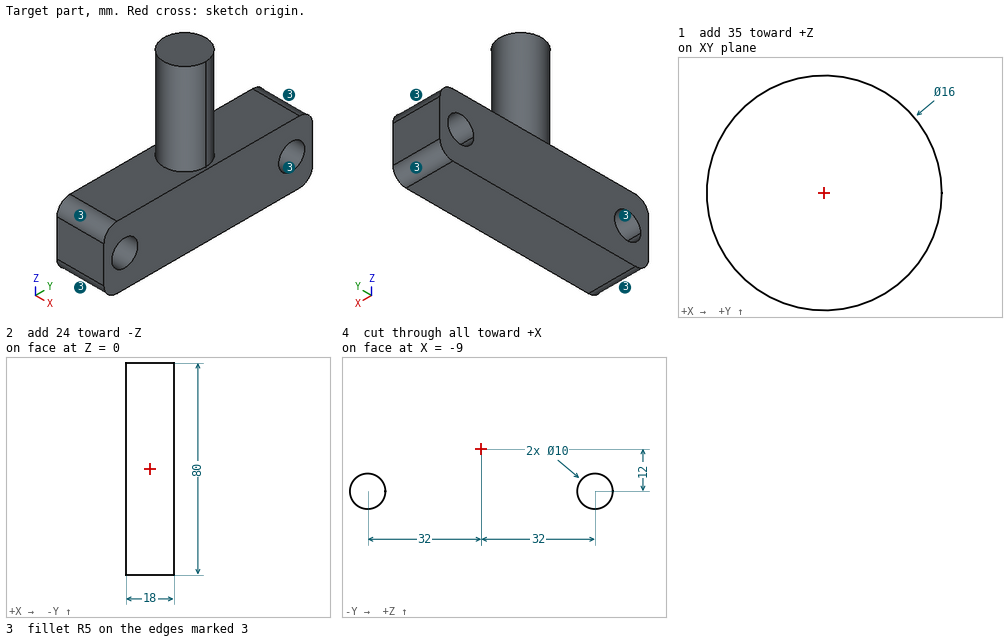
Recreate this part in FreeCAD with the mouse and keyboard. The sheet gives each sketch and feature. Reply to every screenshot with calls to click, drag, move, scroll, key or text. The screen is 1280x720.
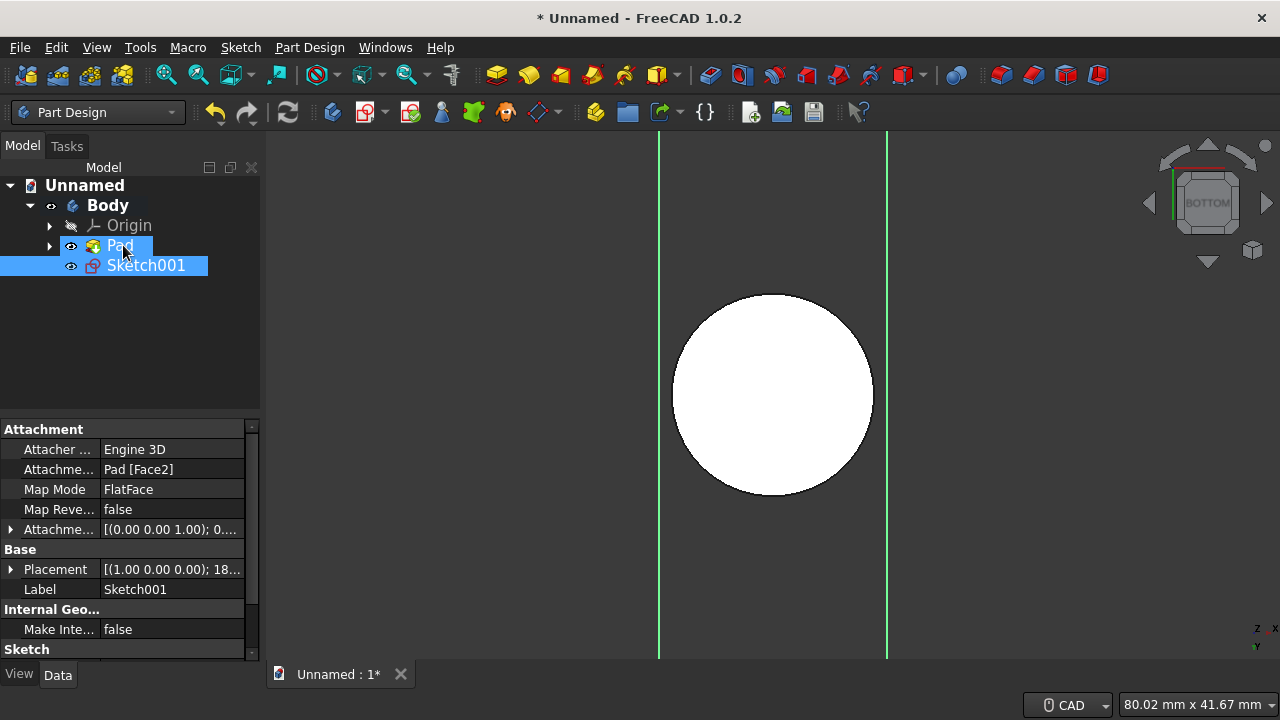
click(498, 76)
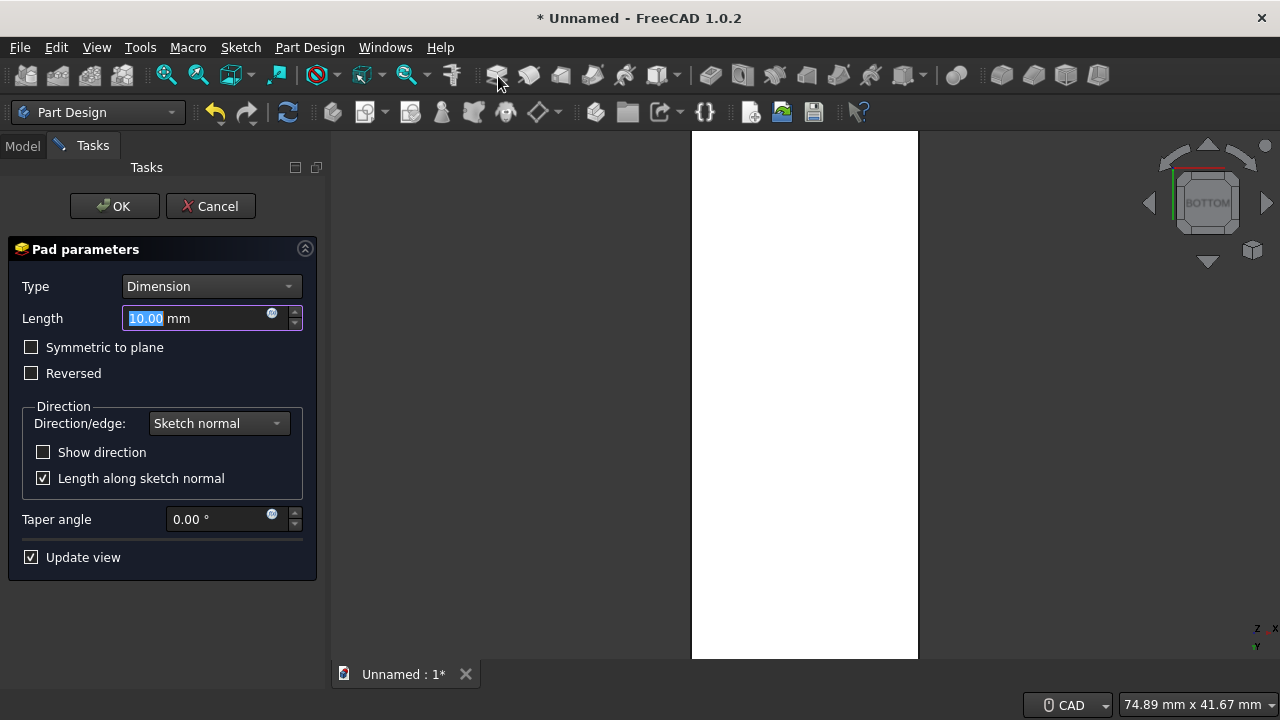
text(24)
key(Tab)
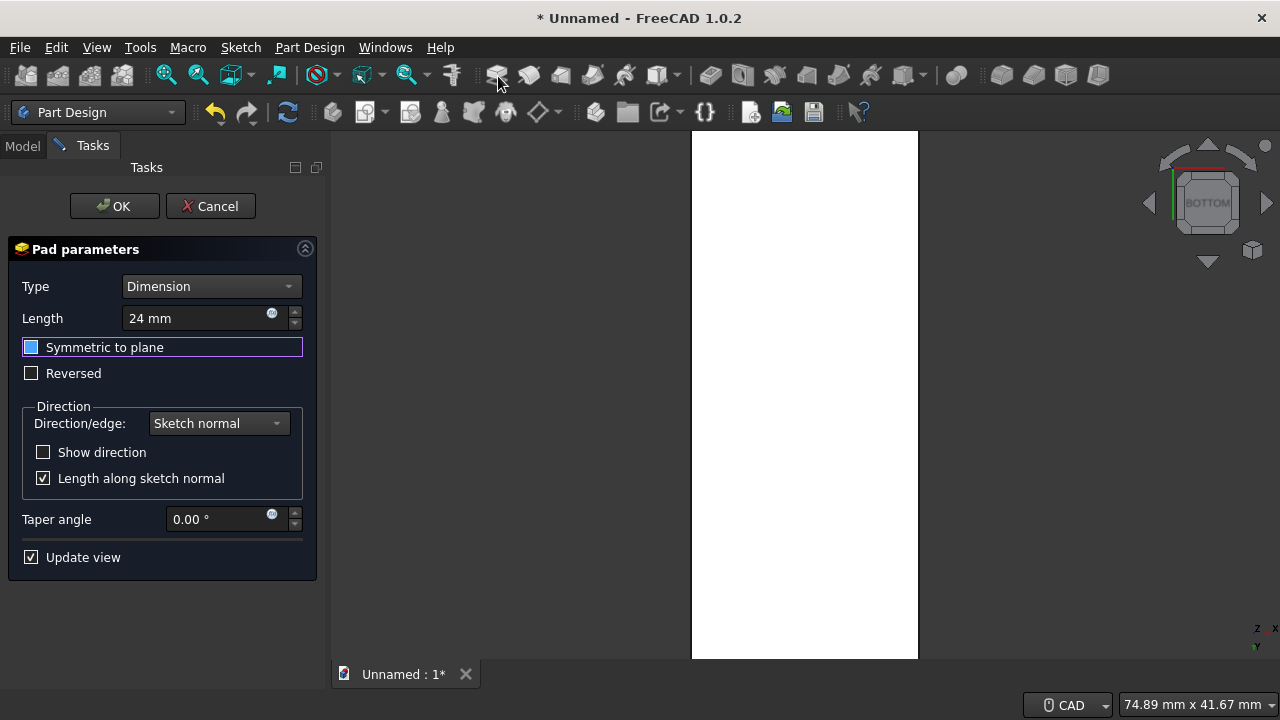
click(115, 206)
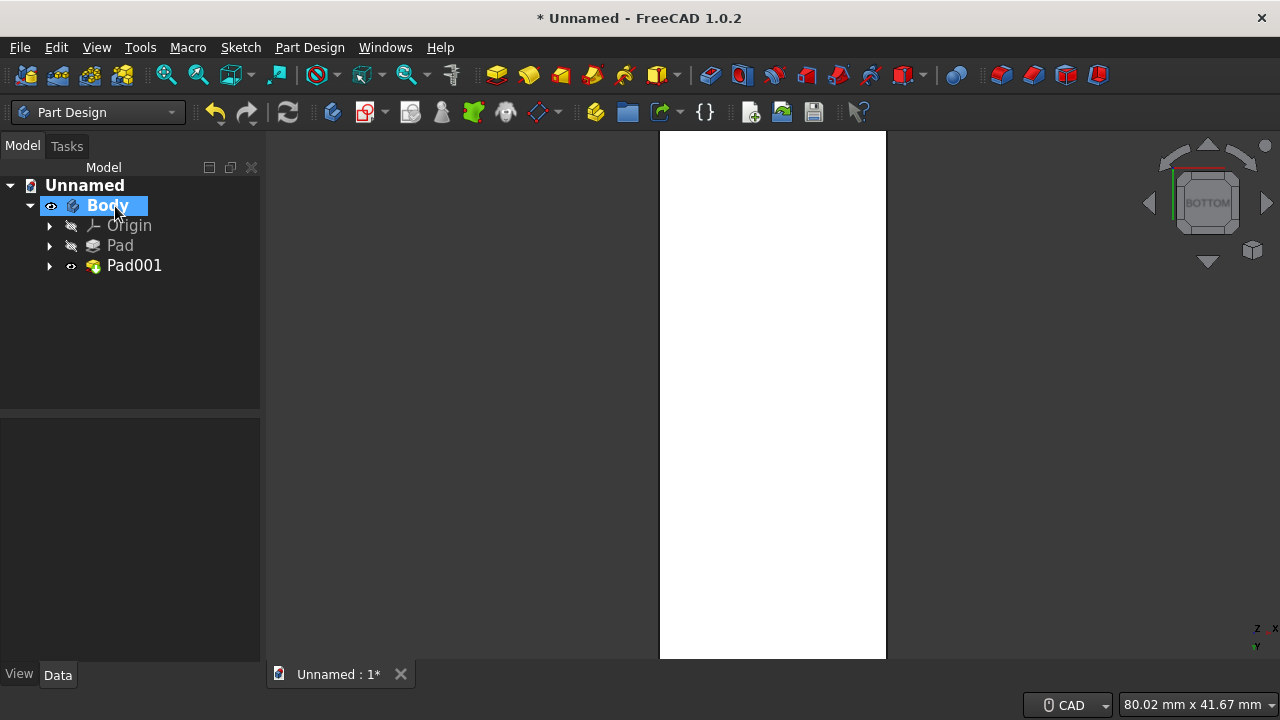
click(168, 76)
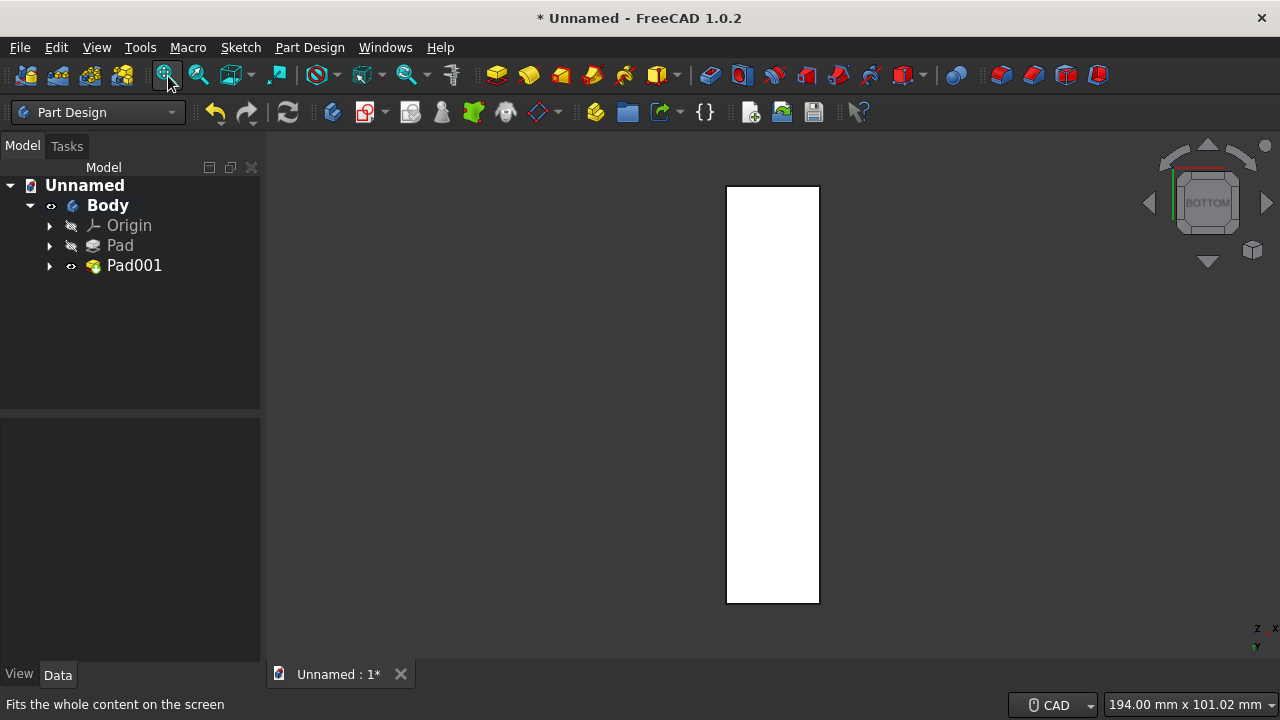
click(773, 603)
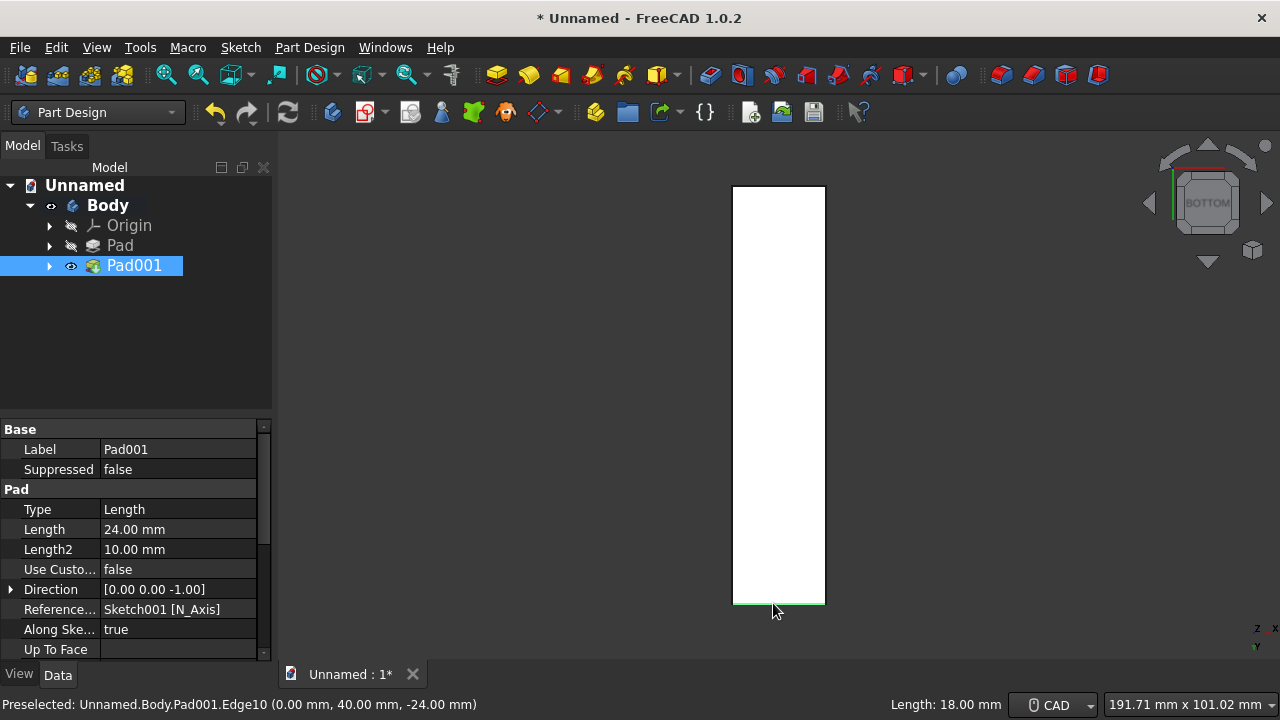
key(0)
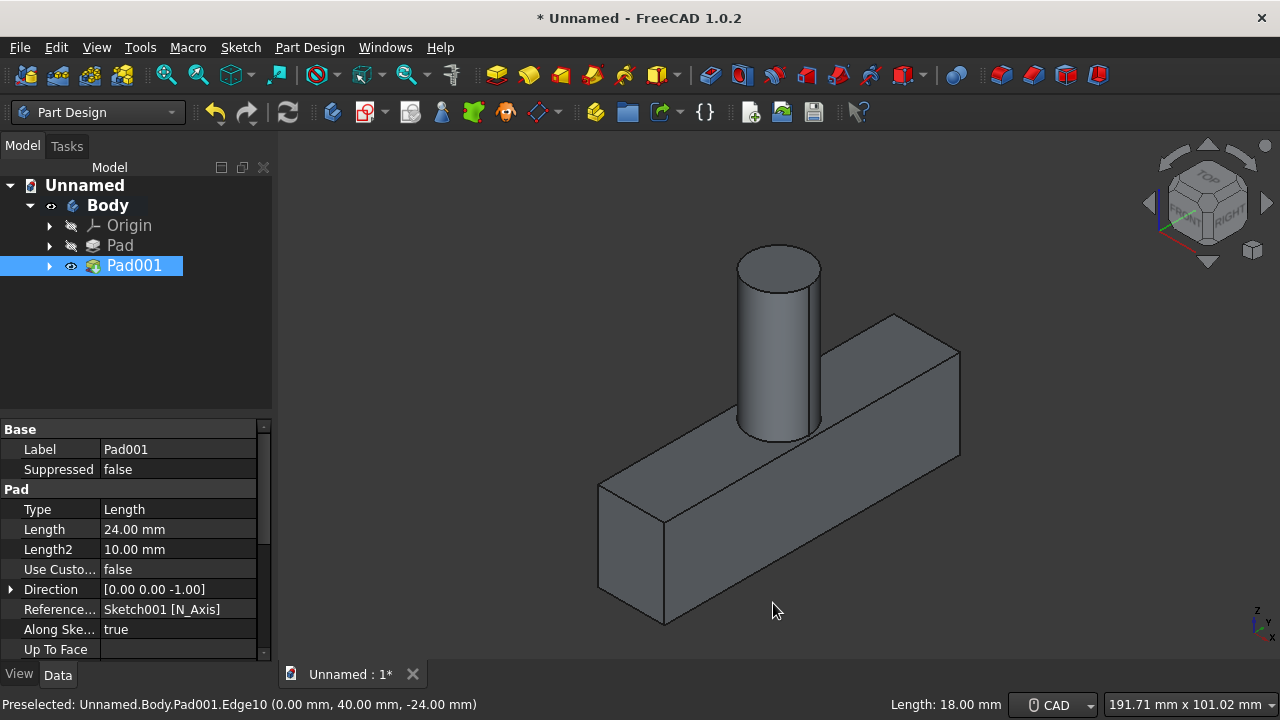
click(631, 503, ctrl)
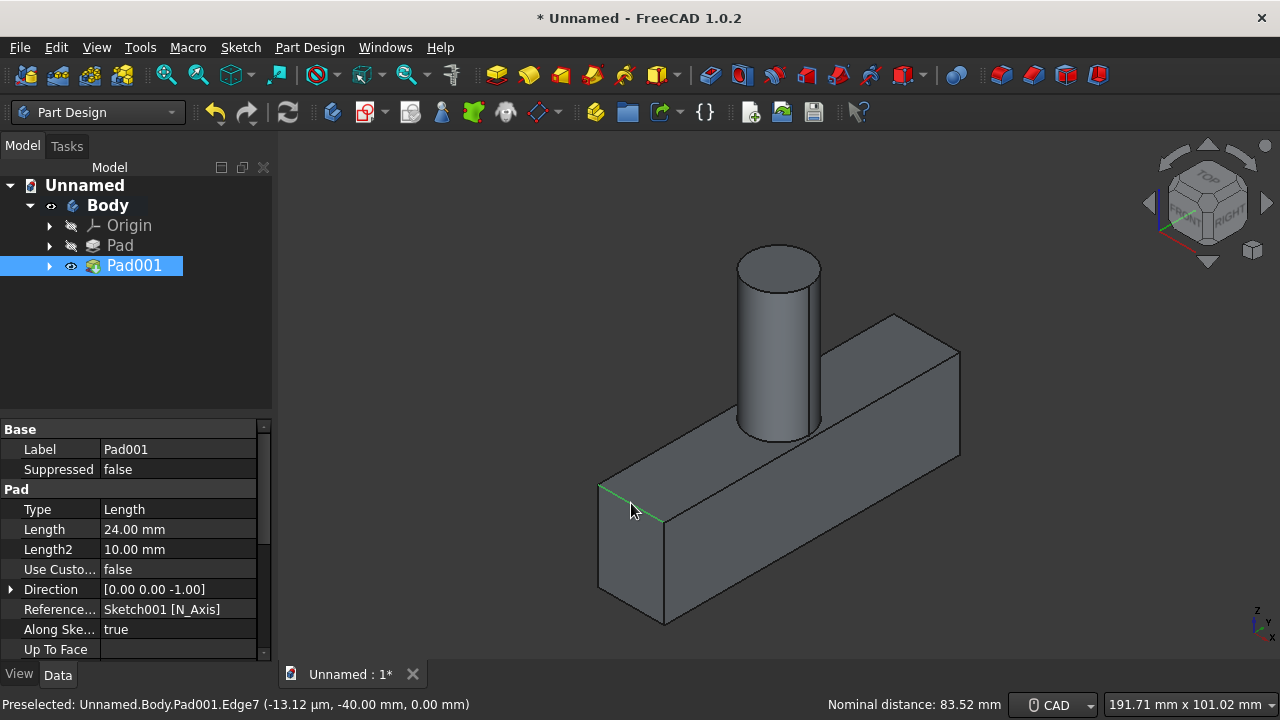
key(2)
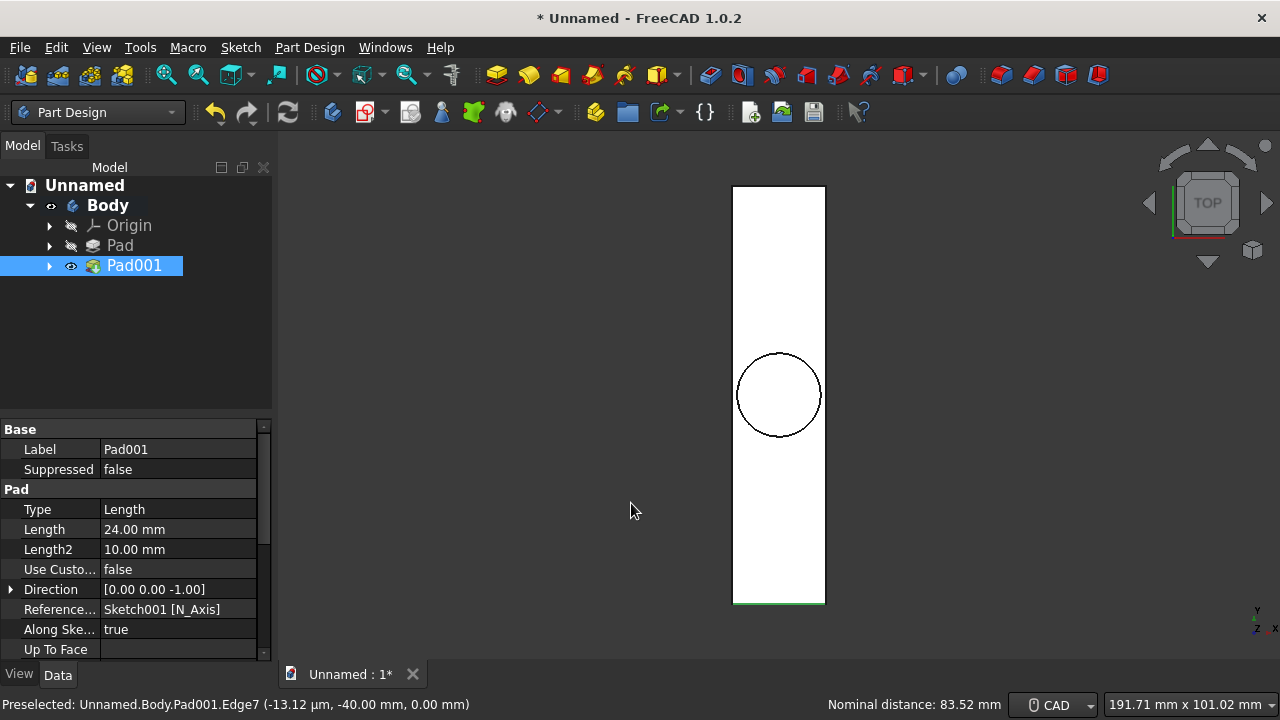
click(779, 185, ctrl)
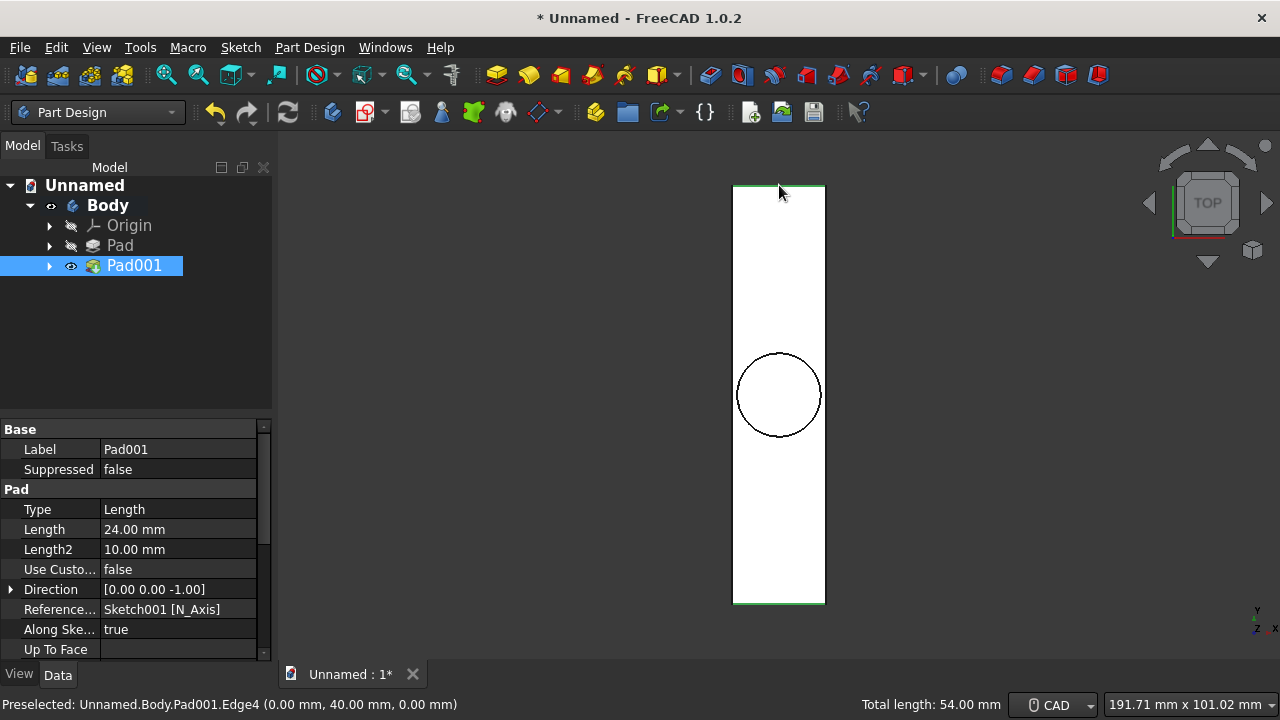
key(1)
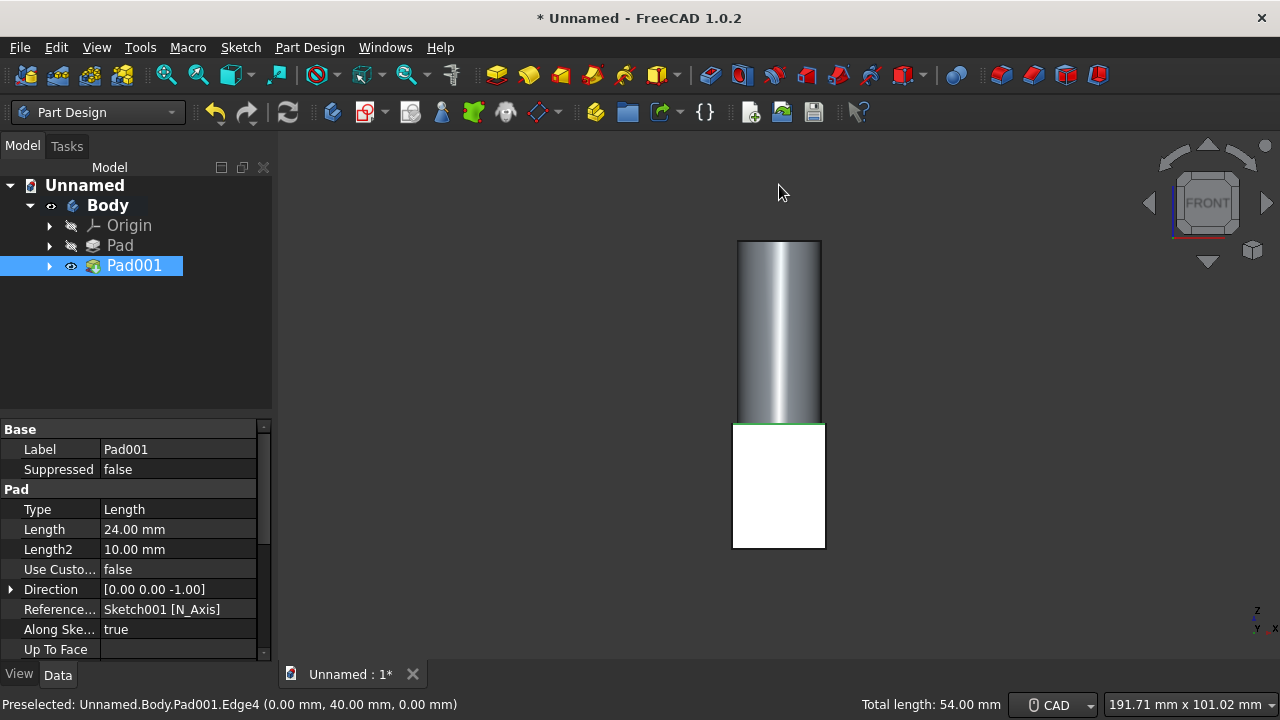
click(779, 548, ctrl)